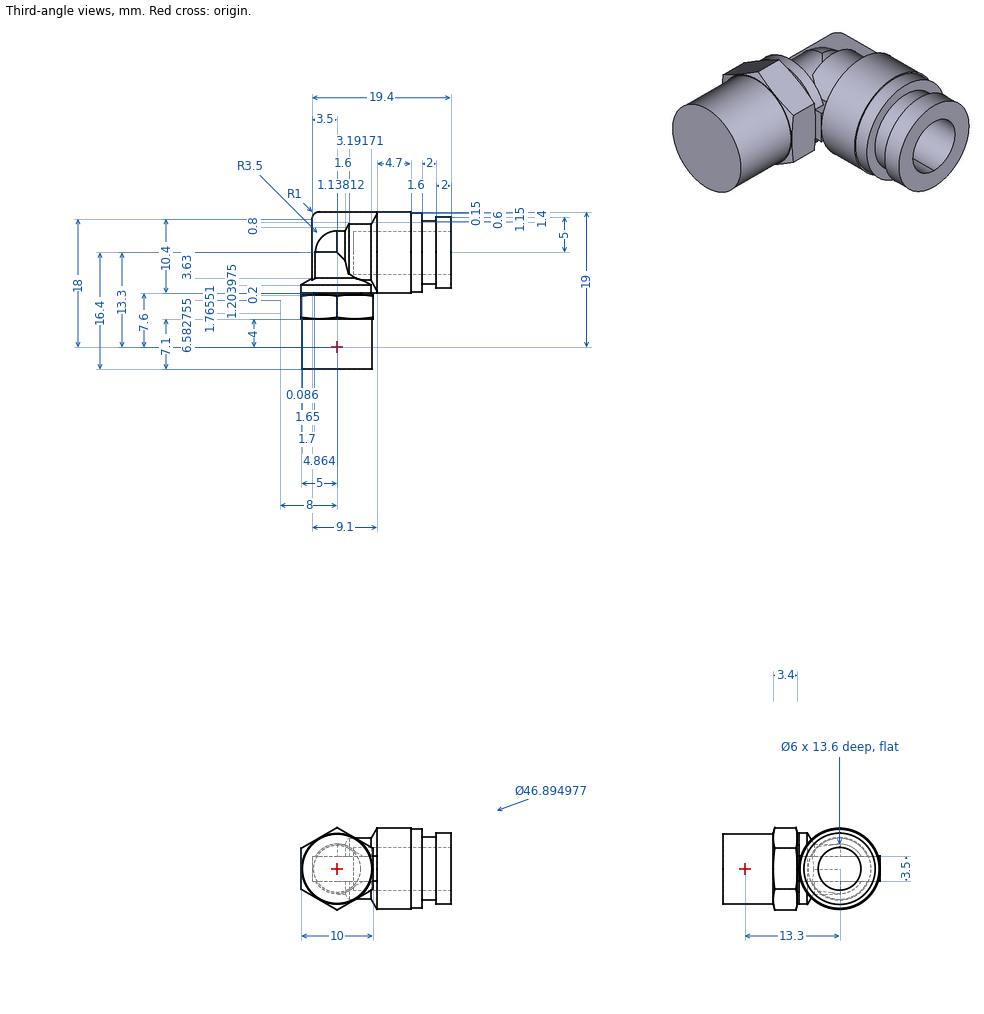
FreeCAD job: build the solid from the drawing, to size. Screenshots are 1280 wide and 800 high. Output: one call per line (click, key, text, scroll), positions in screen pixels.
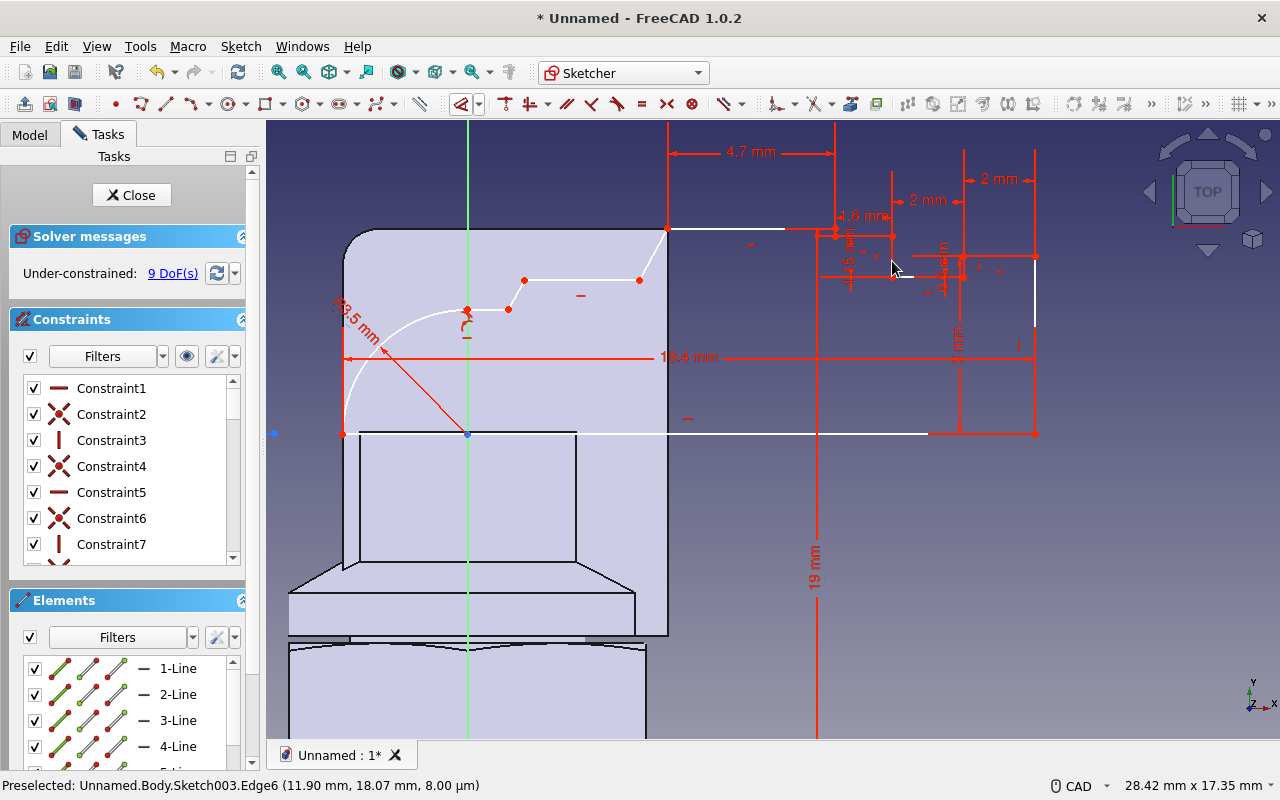
scroll(835, 233, up, 11)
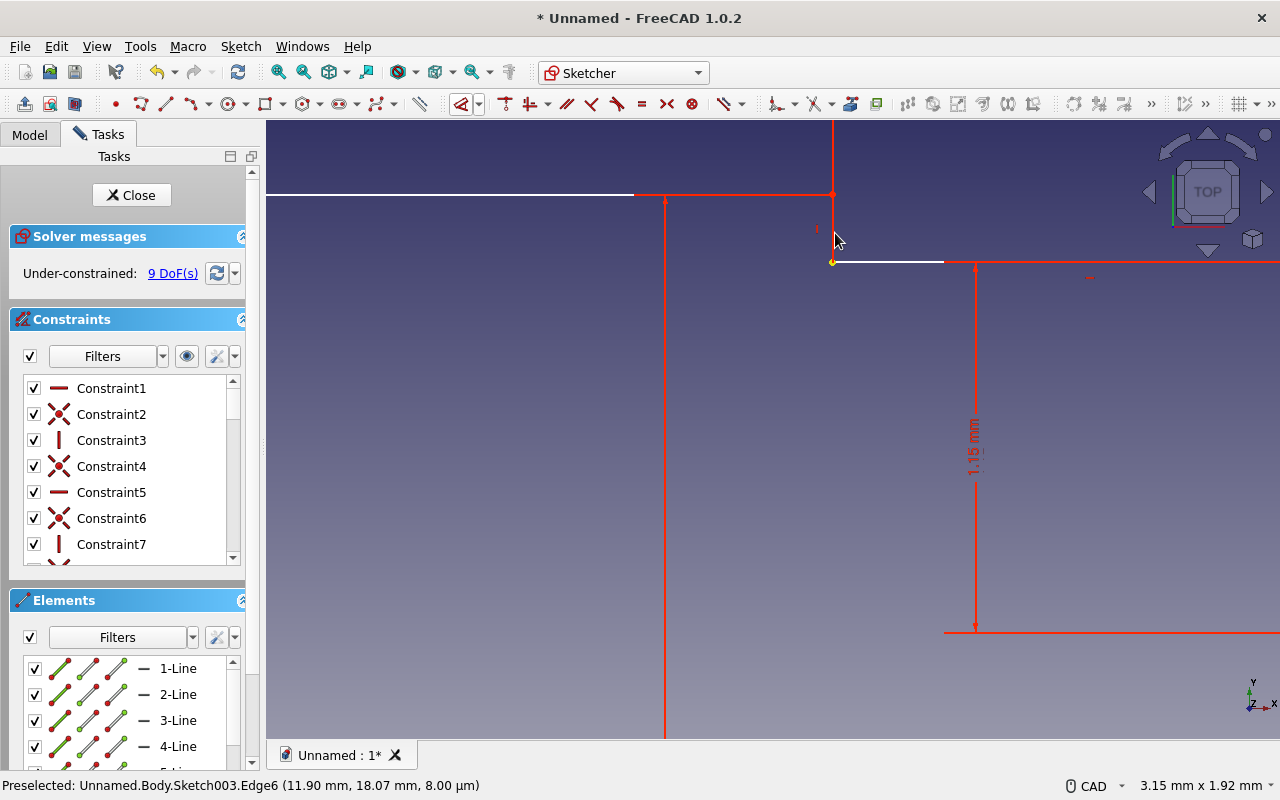
click(833, 228)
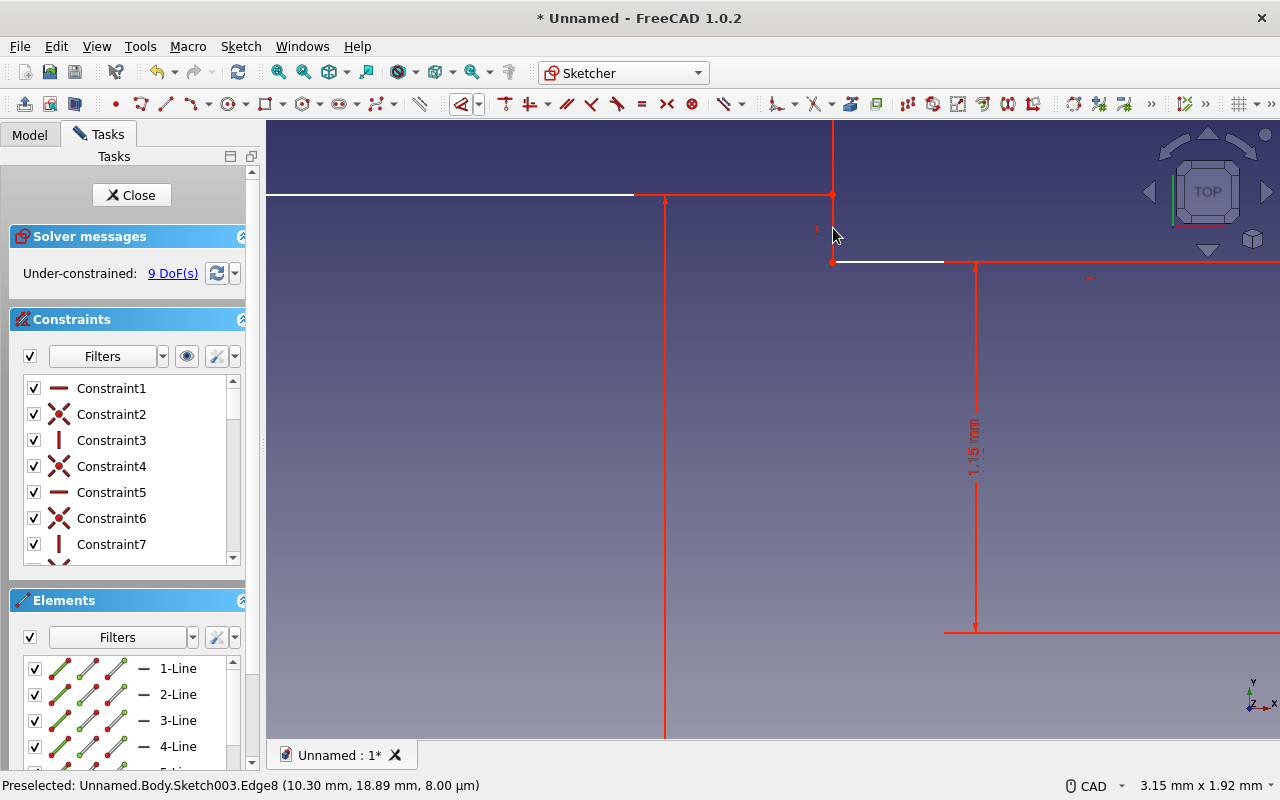
key(i)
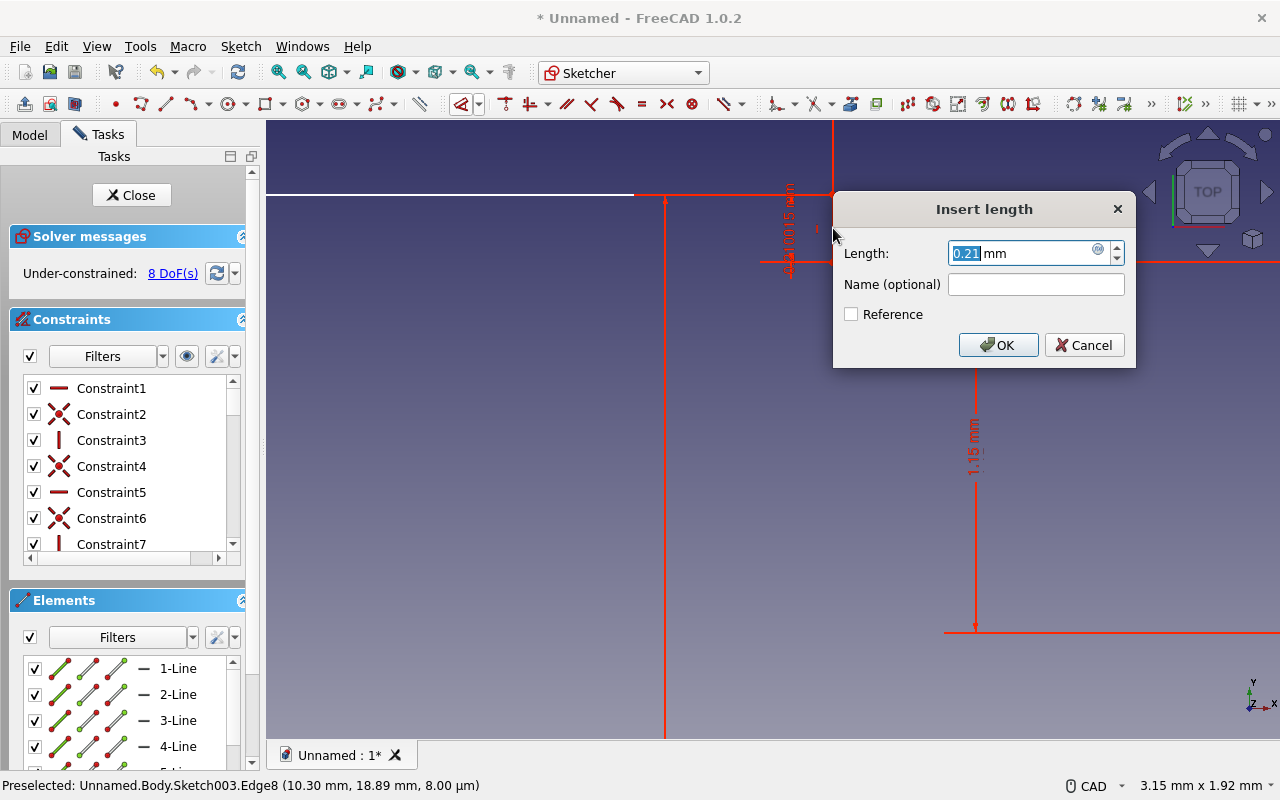
text(0.15)
key(Return)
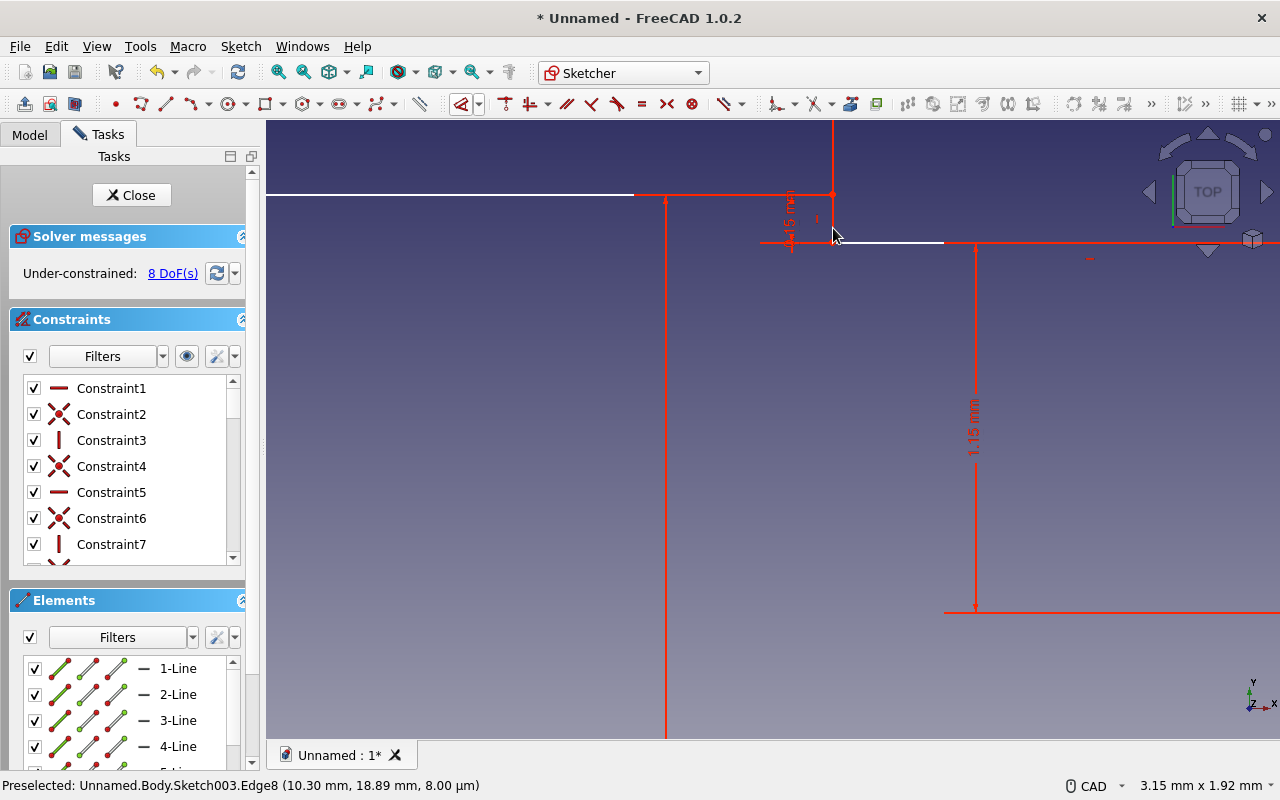
scroll(863, 247, down, 14)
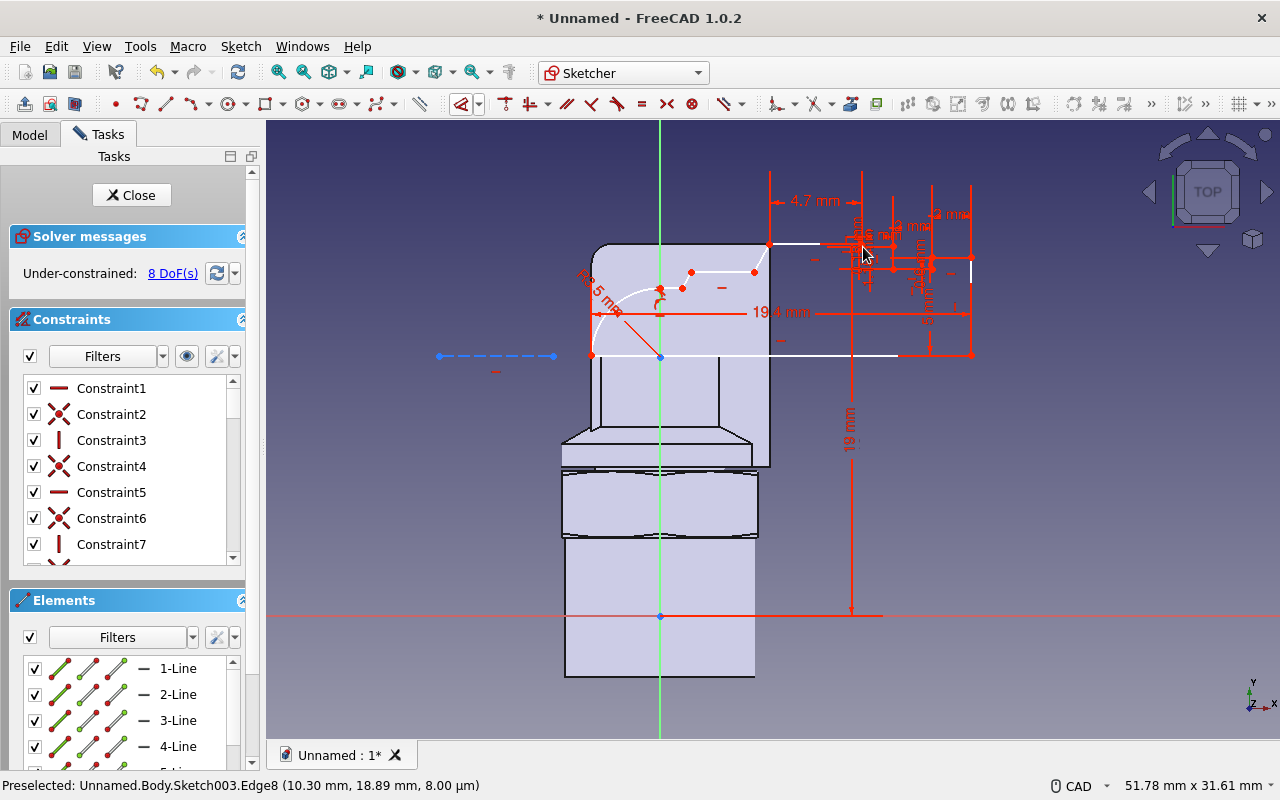
scroll(691, 272, up, 2)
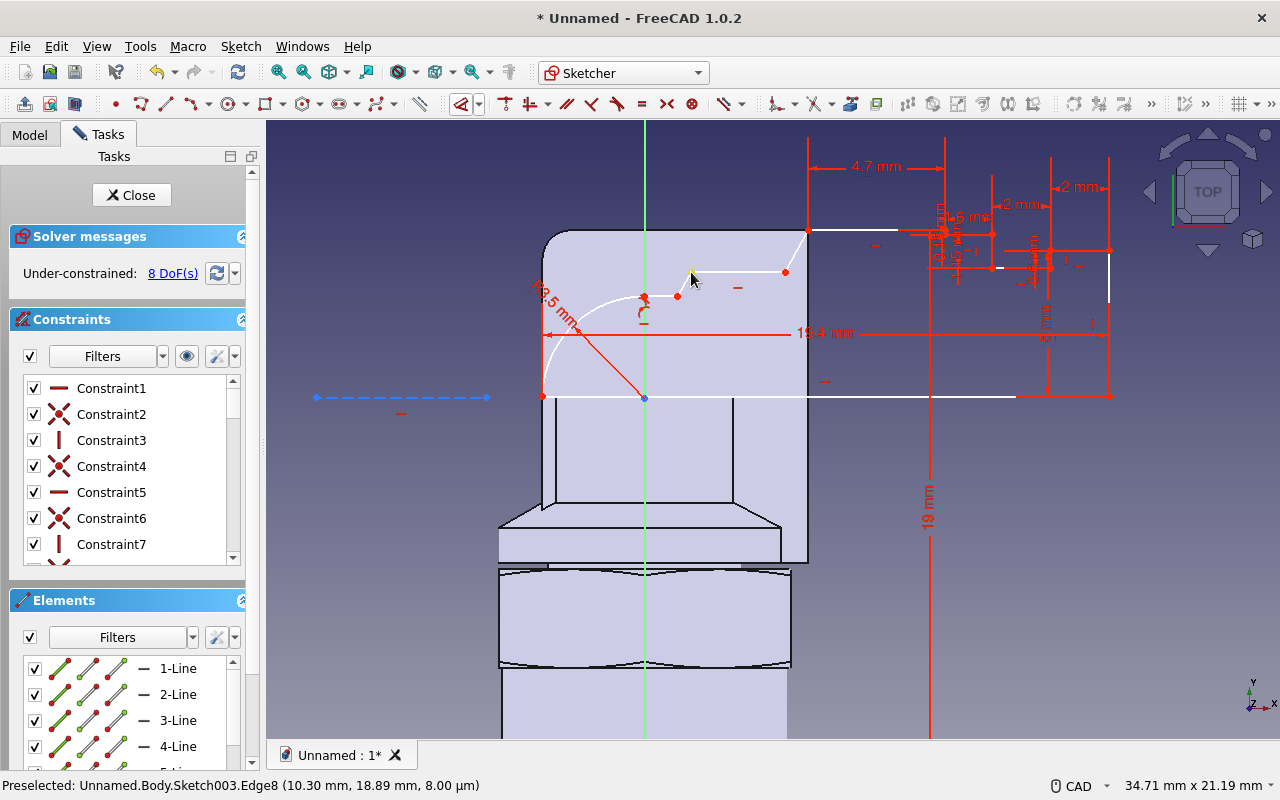
click(691, 272)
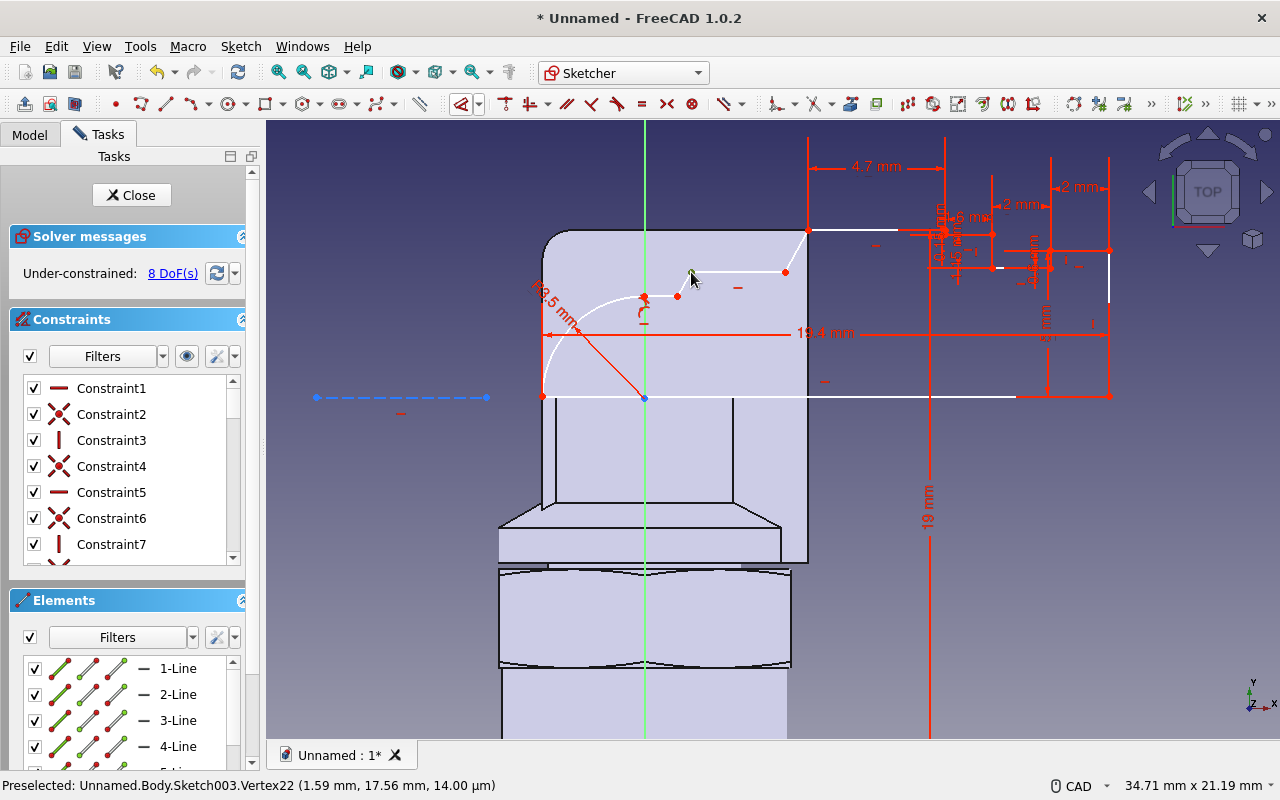
key(l)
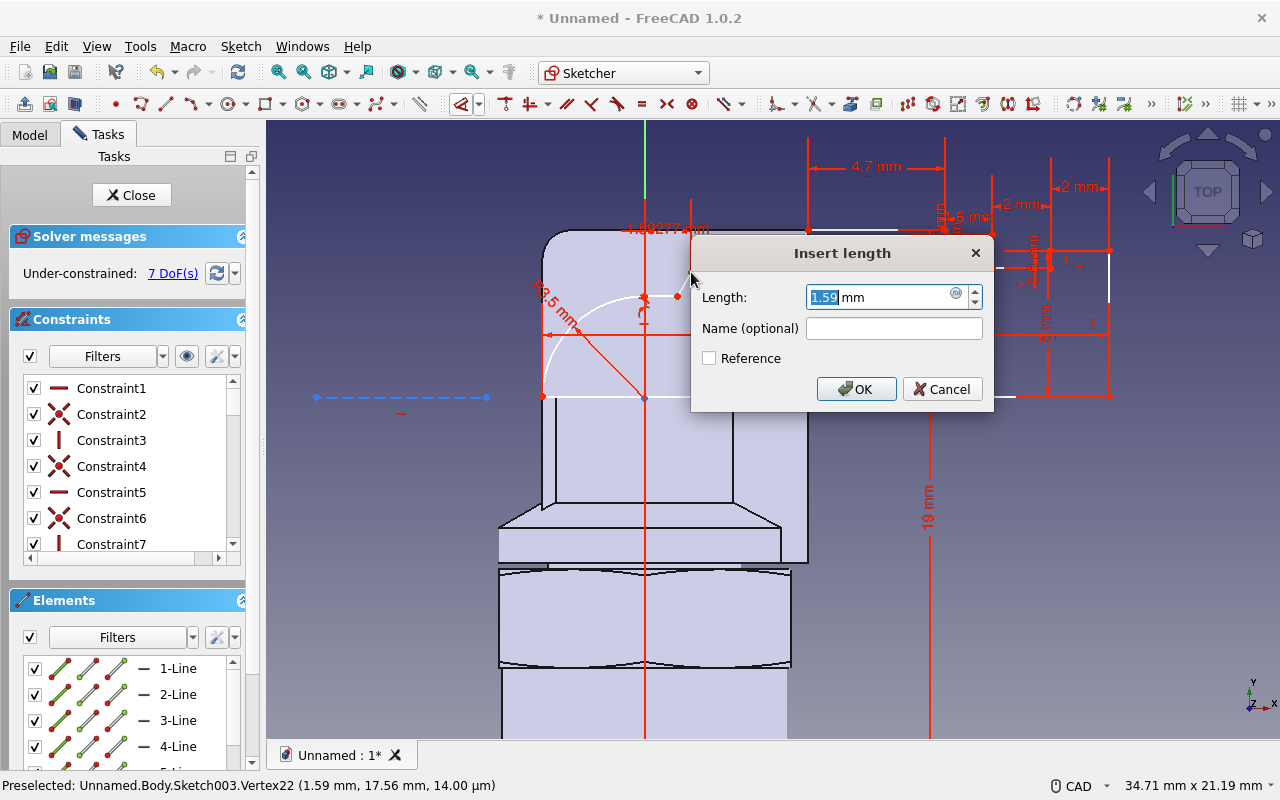
text(1.6)
key(Return)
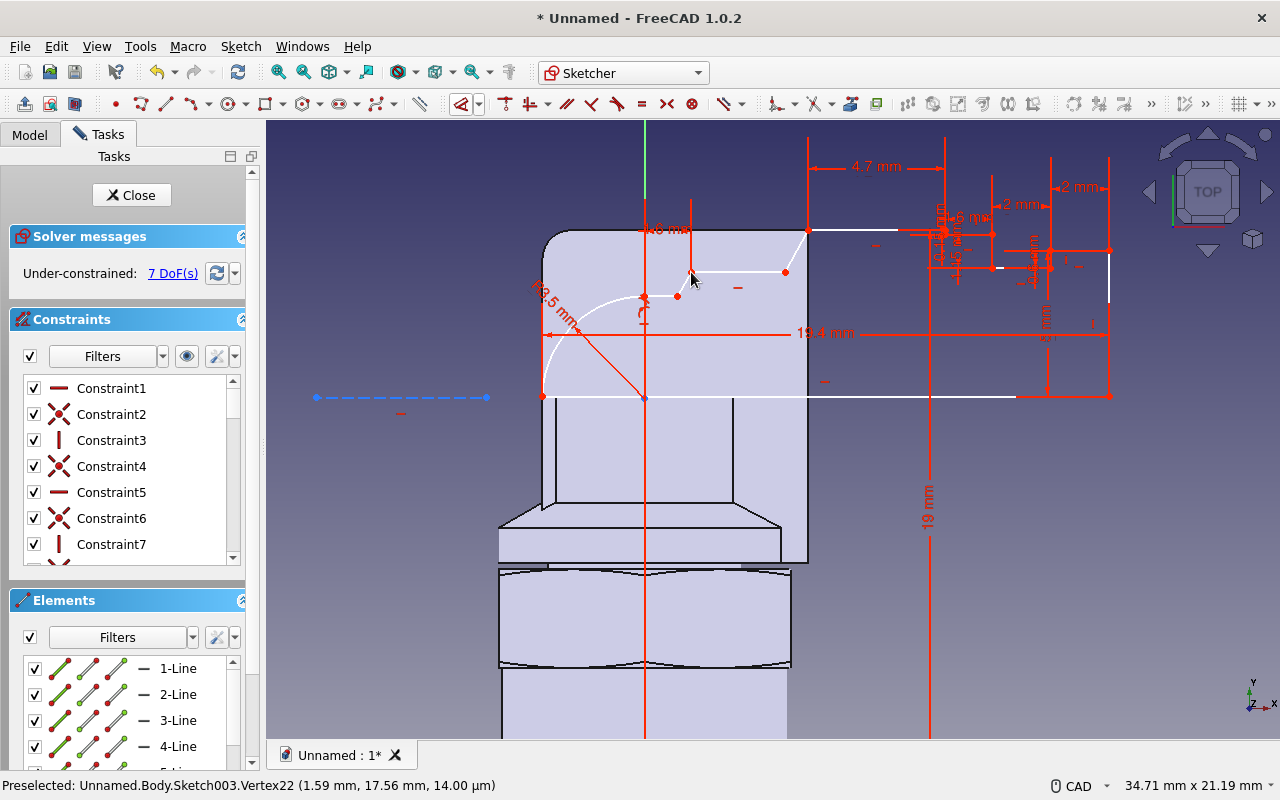
click(801, 243)